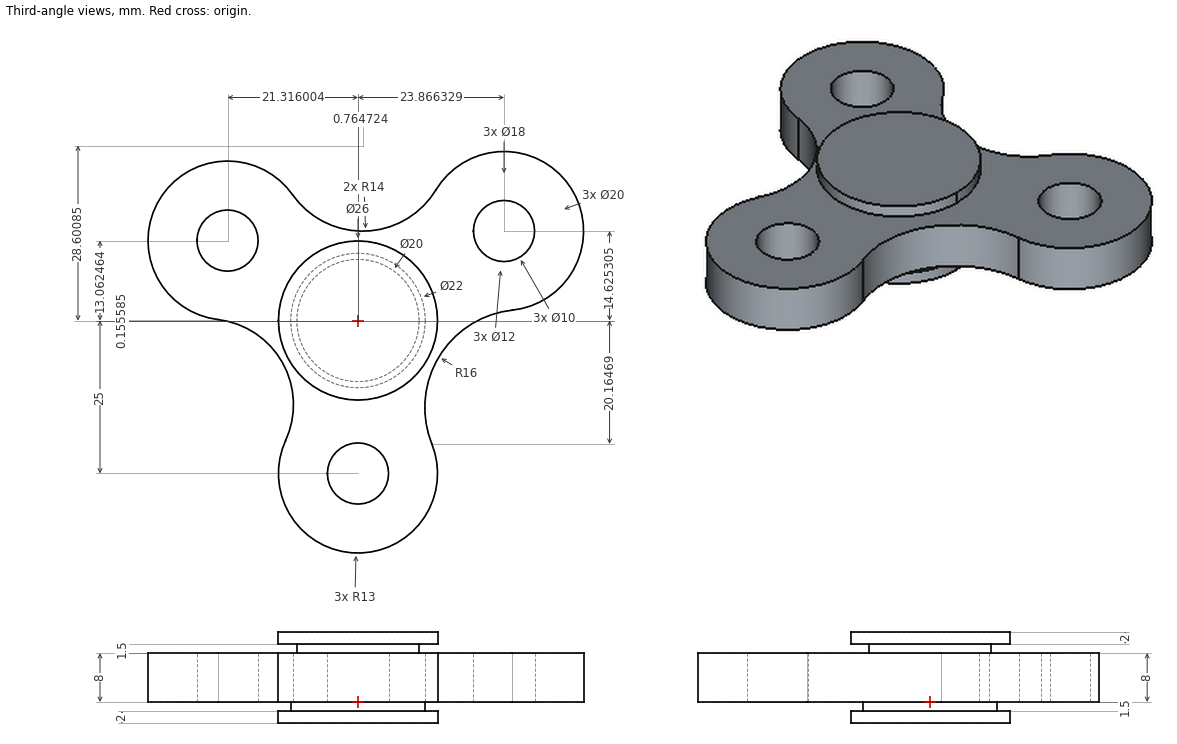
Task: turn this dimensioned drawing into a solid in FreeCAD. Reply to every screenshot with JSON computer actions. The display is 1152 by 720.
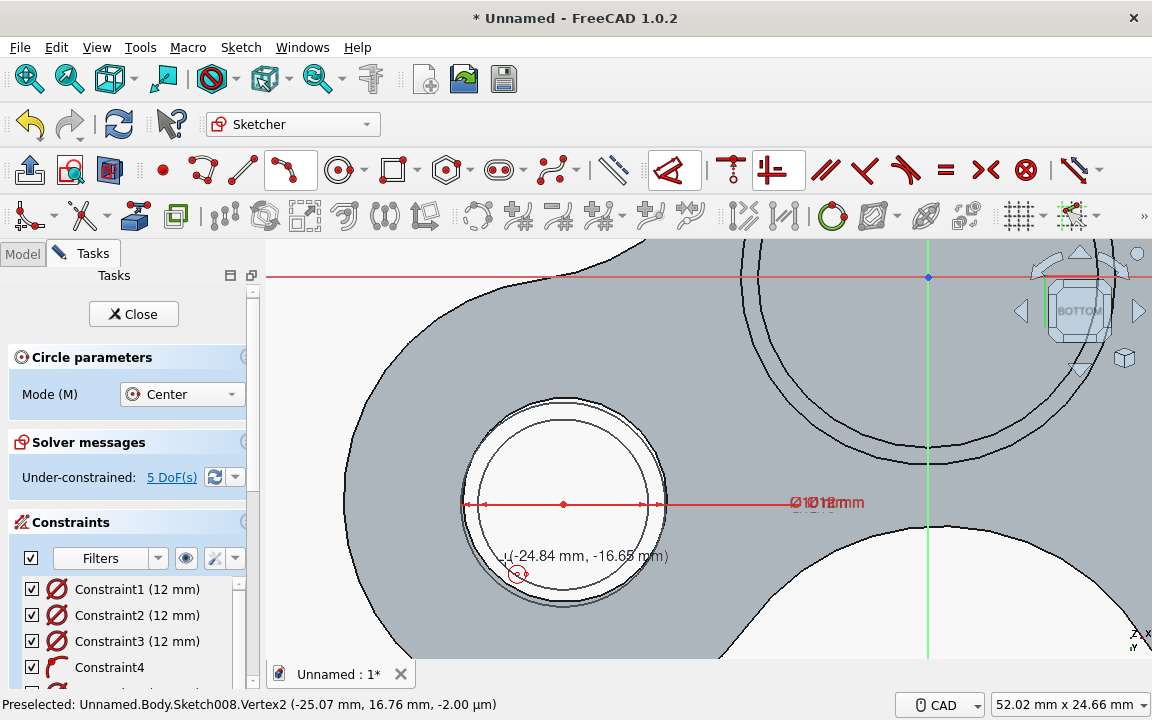
{"action": "scroll", "coordinate": [507, 561], "scroll_direction": "down", "scroll_amount": 6}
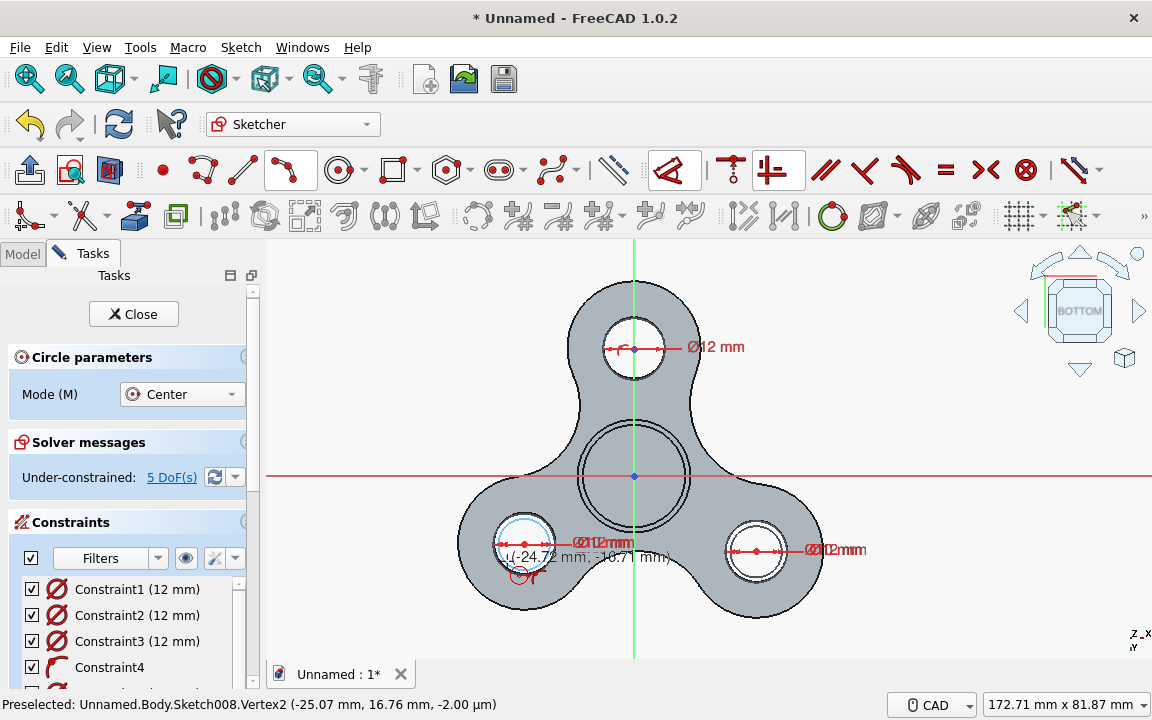
{"action": "left_click", "coordinate": [634, 349]}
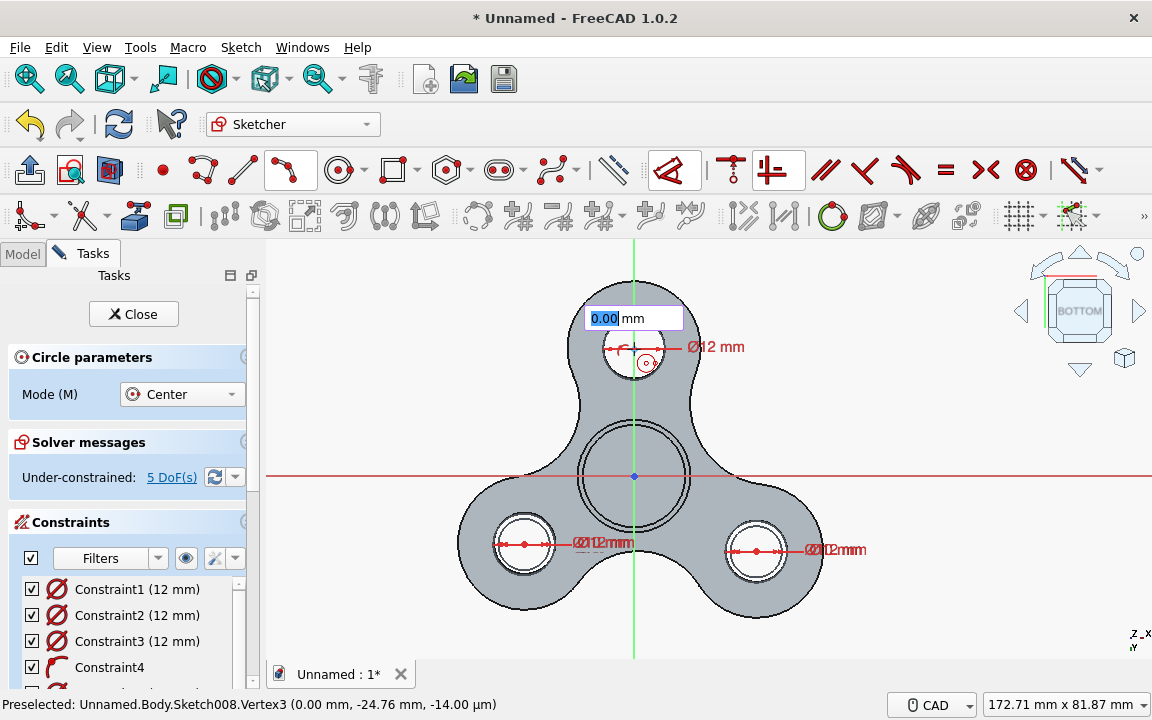
{"action": "scroll", "coordinate": [625, 372], "scroll_direction": "up", "scroll_amount": 6}
{"action": "mouse_move", "coordinate": [625, 371]}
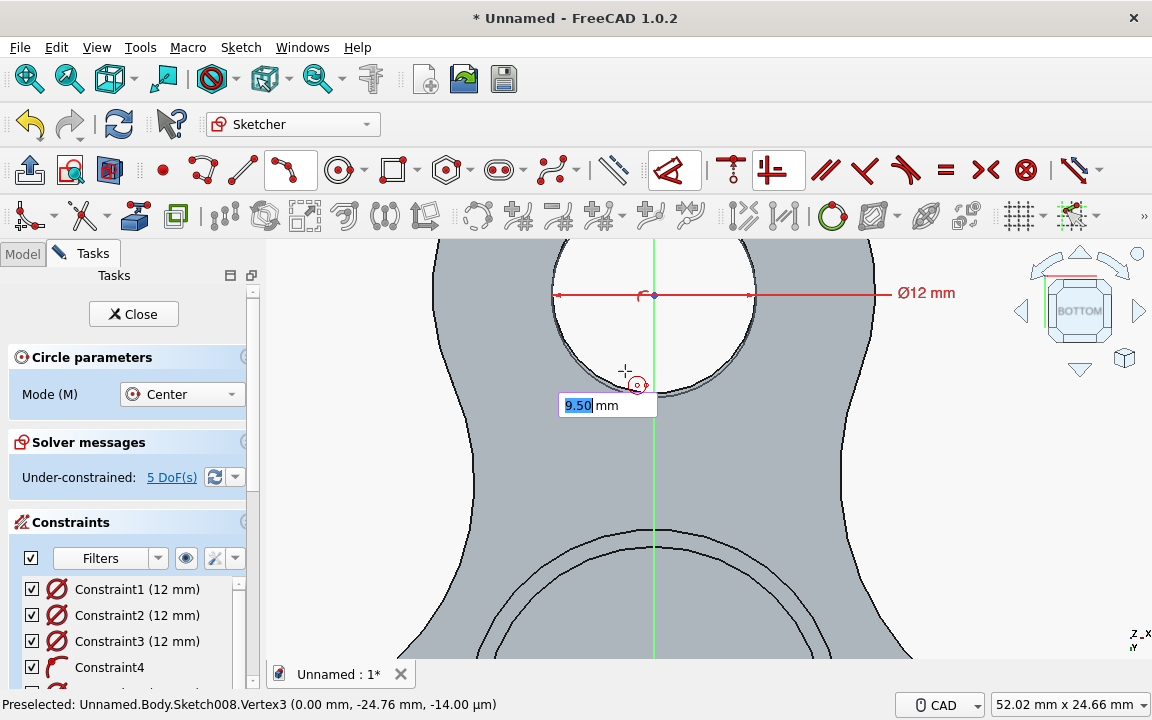
{"action": "type", "text": "10"}
{"action": "key", "text": "Return"}
{"action": "key", "text": "Escape"}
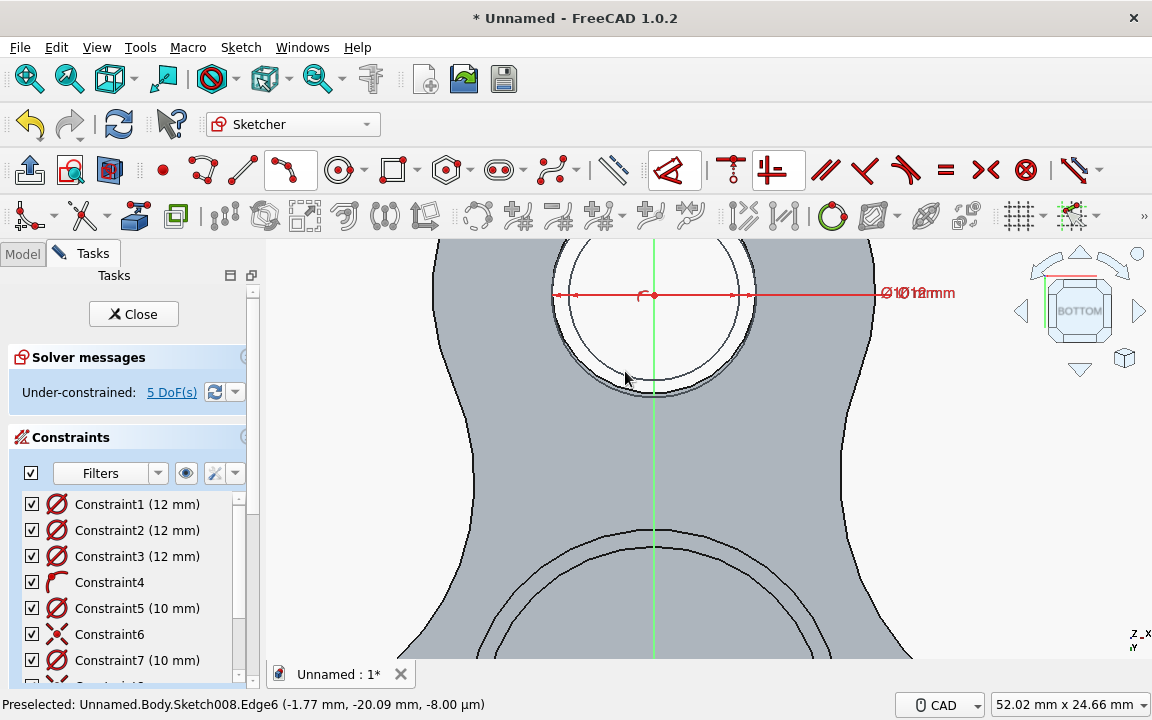
{"action": "scroll", "coordinate": [625, 372], "scroll_direction": "down", "scroll_amount": 6}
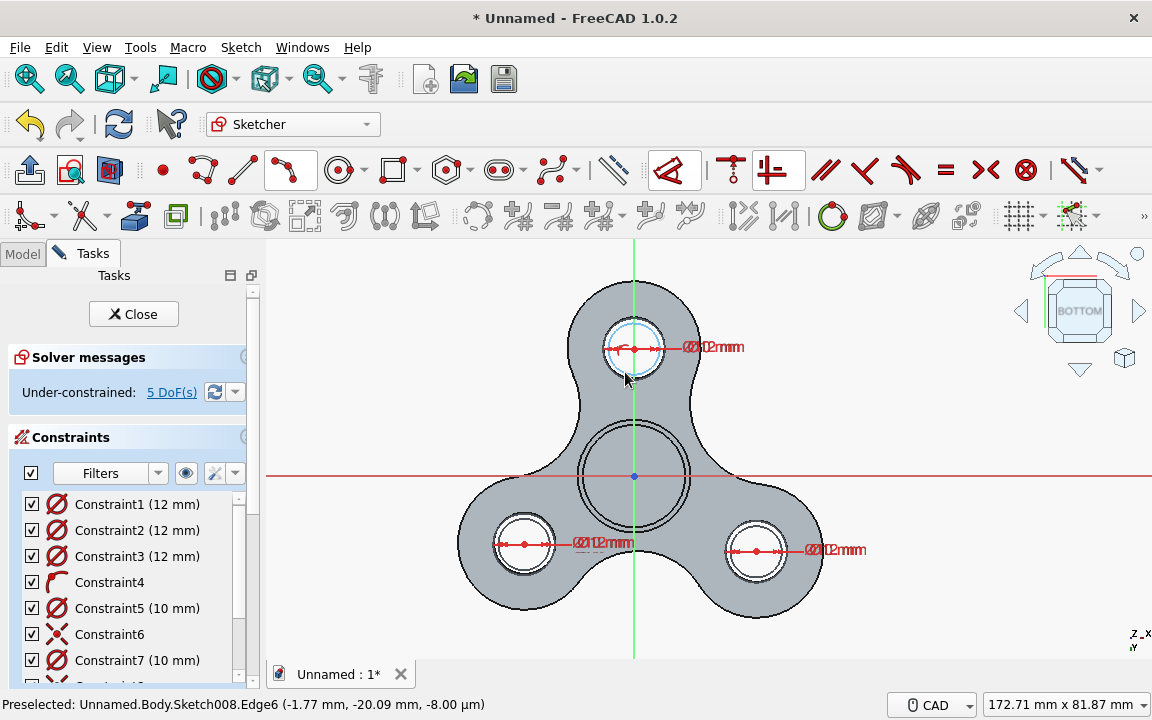
{"action": "left_click", "coordinate": [634, 349]}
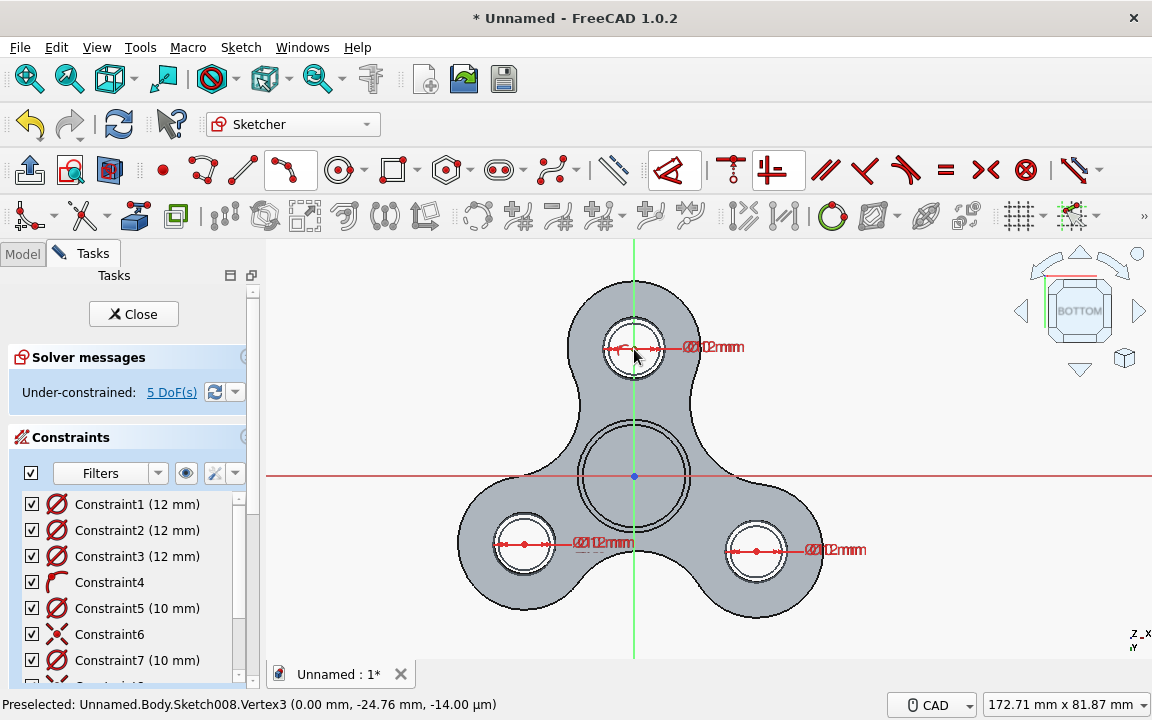
{"action": "key", "text": "i"}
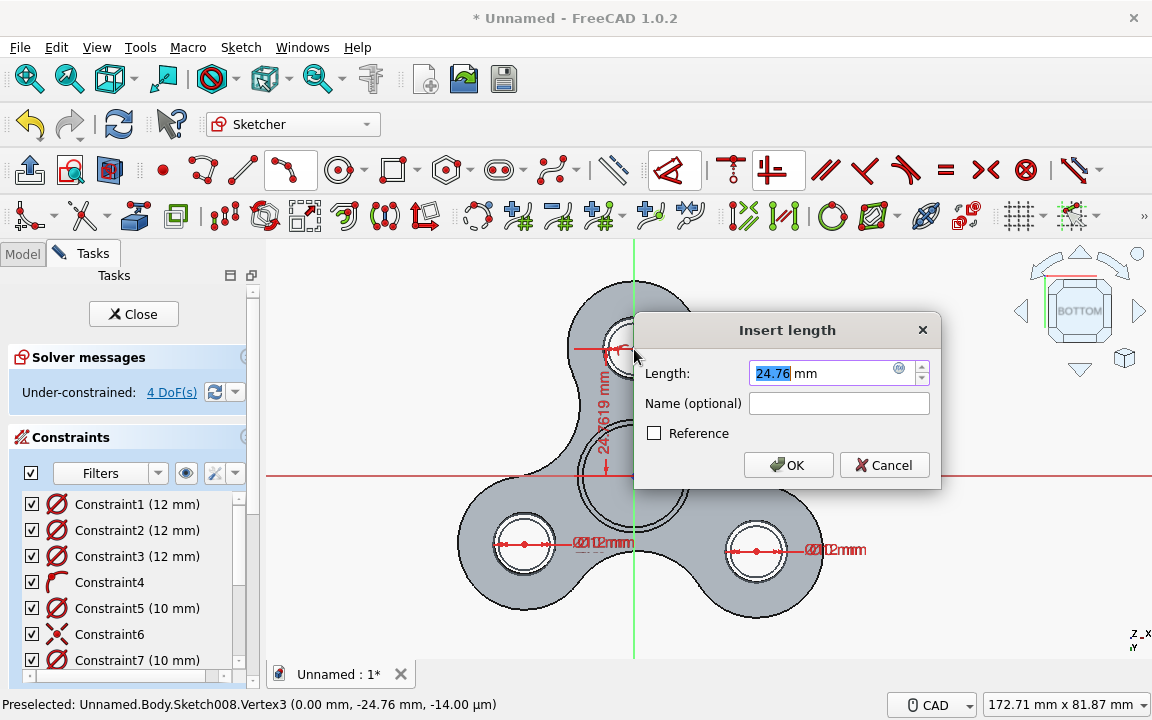
{"action": "type", "text": "25"}
{"action": "key", "text": "Return"}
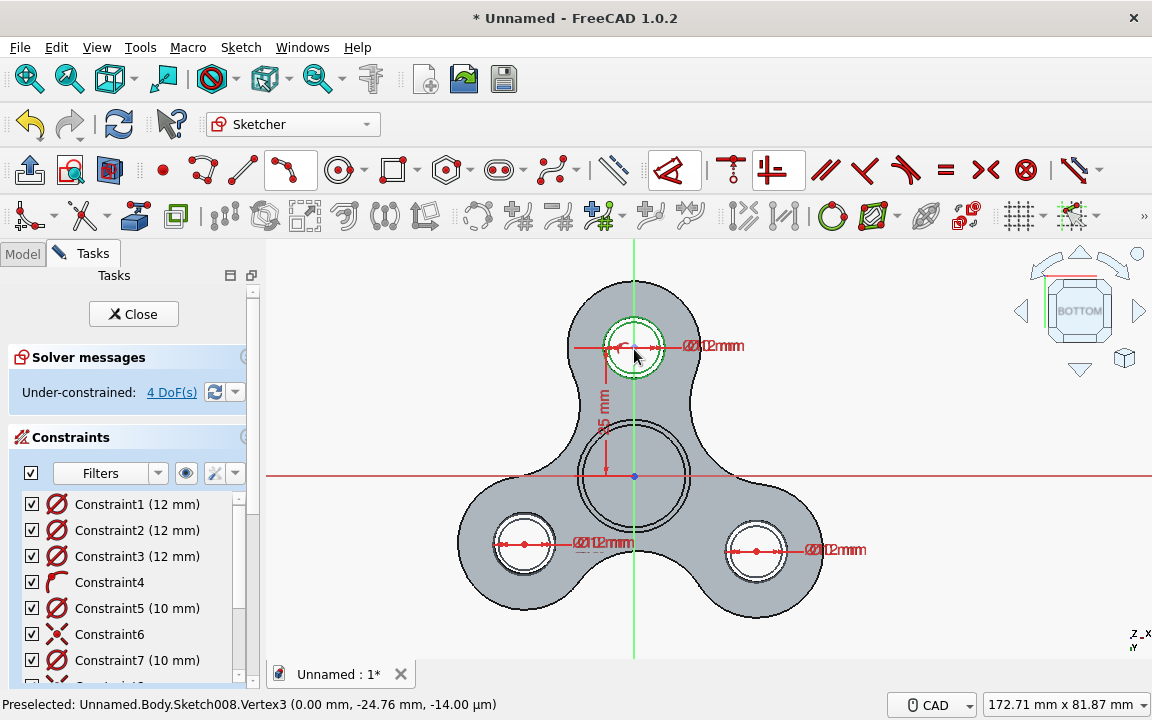
{"action": "left_click", "coordinate": [756, 552]}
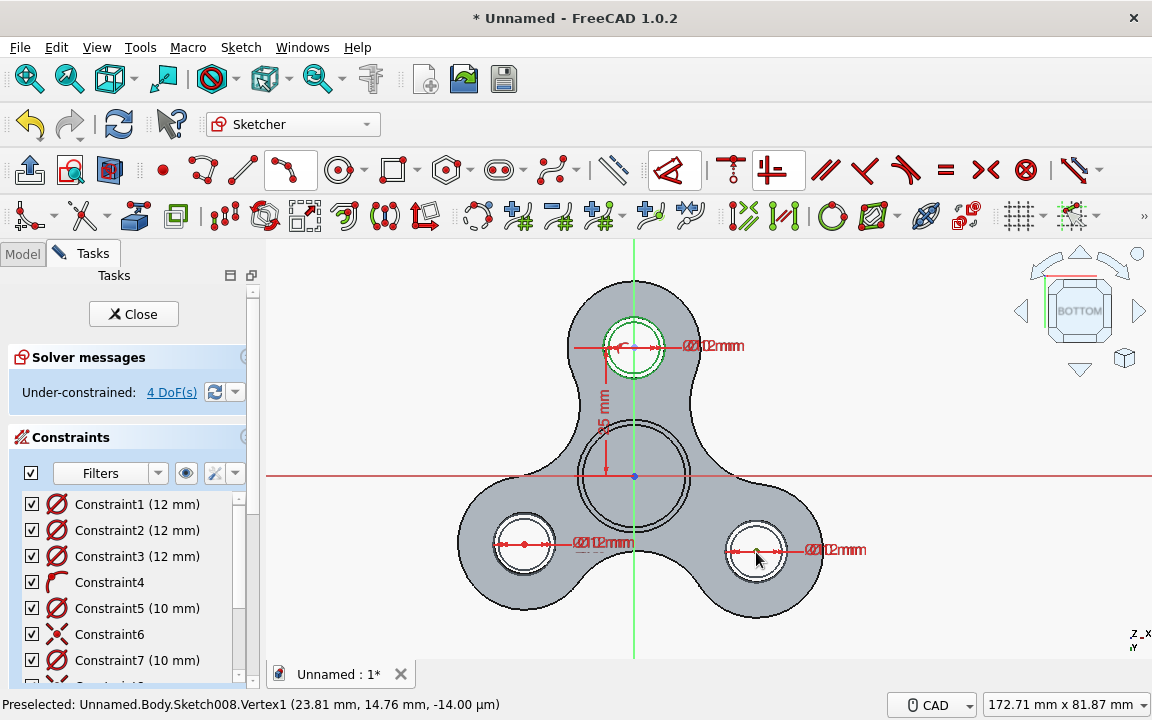
{"action": "key", "text": "l"}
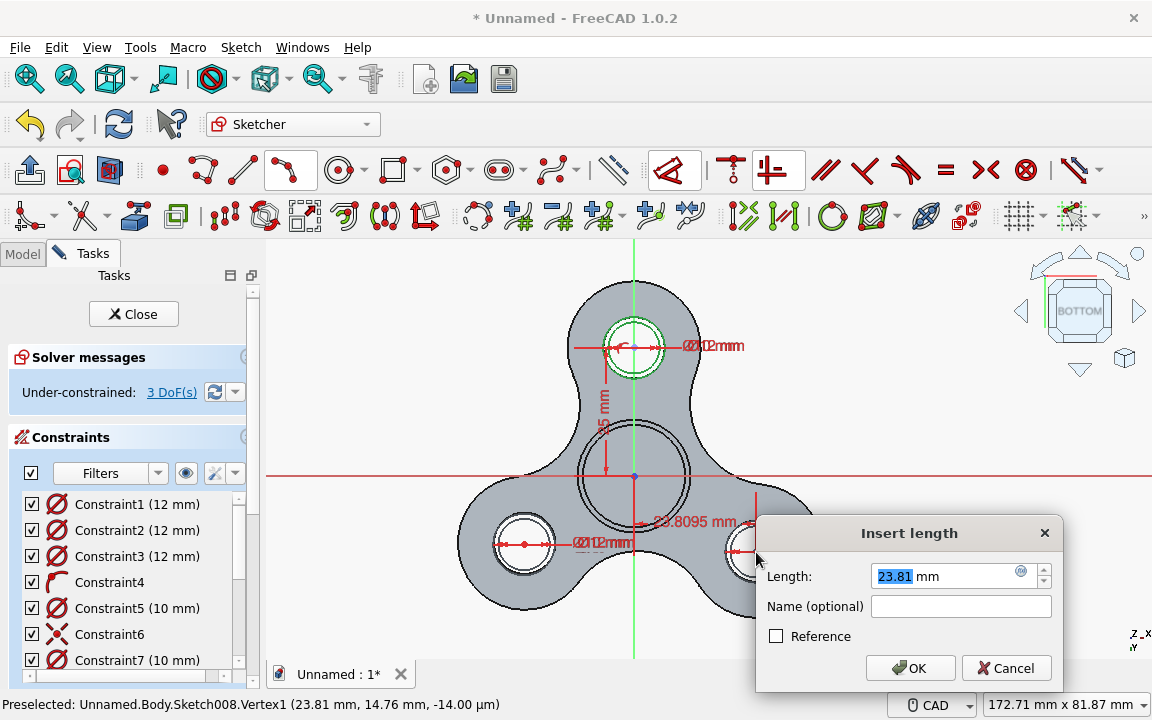
{"action": "type", "text": "23.866329"}
{"action": "key", "text": "Return"}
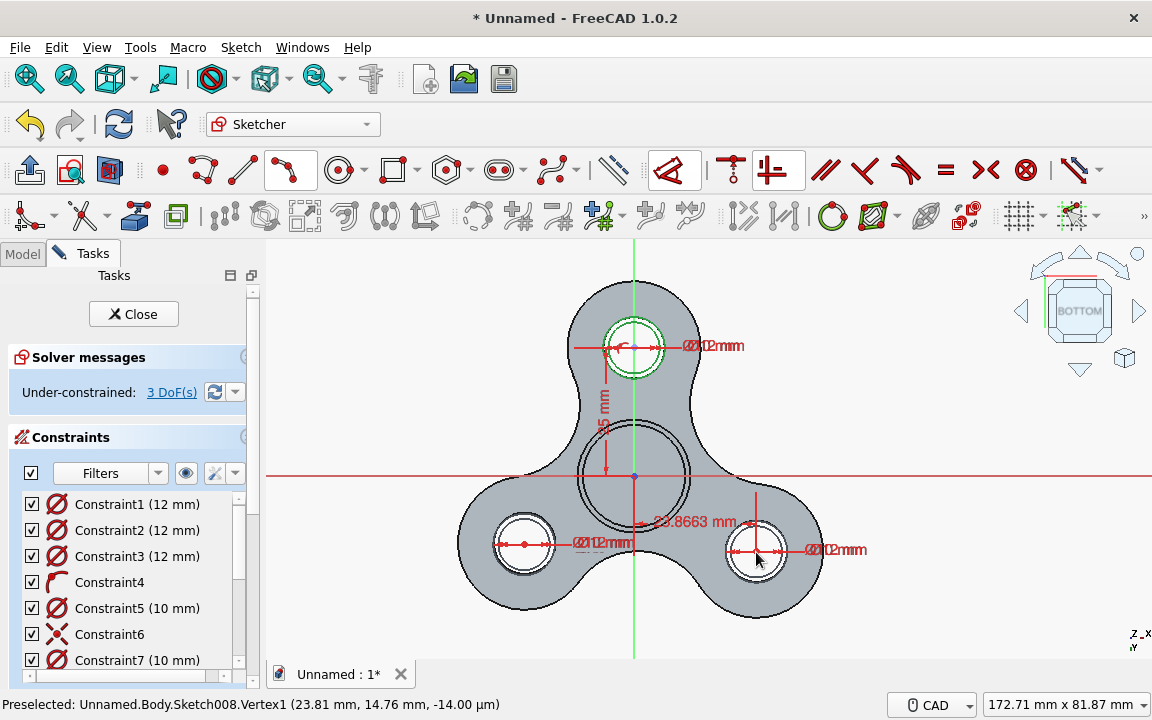
{"action": "left_click", "coordinate": [756, 552]}